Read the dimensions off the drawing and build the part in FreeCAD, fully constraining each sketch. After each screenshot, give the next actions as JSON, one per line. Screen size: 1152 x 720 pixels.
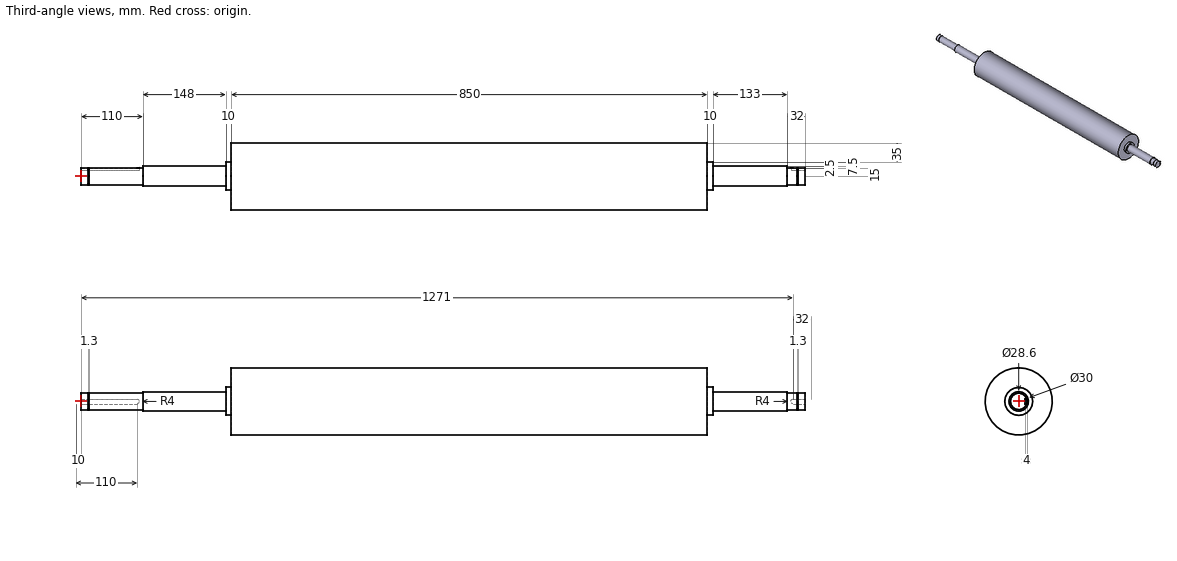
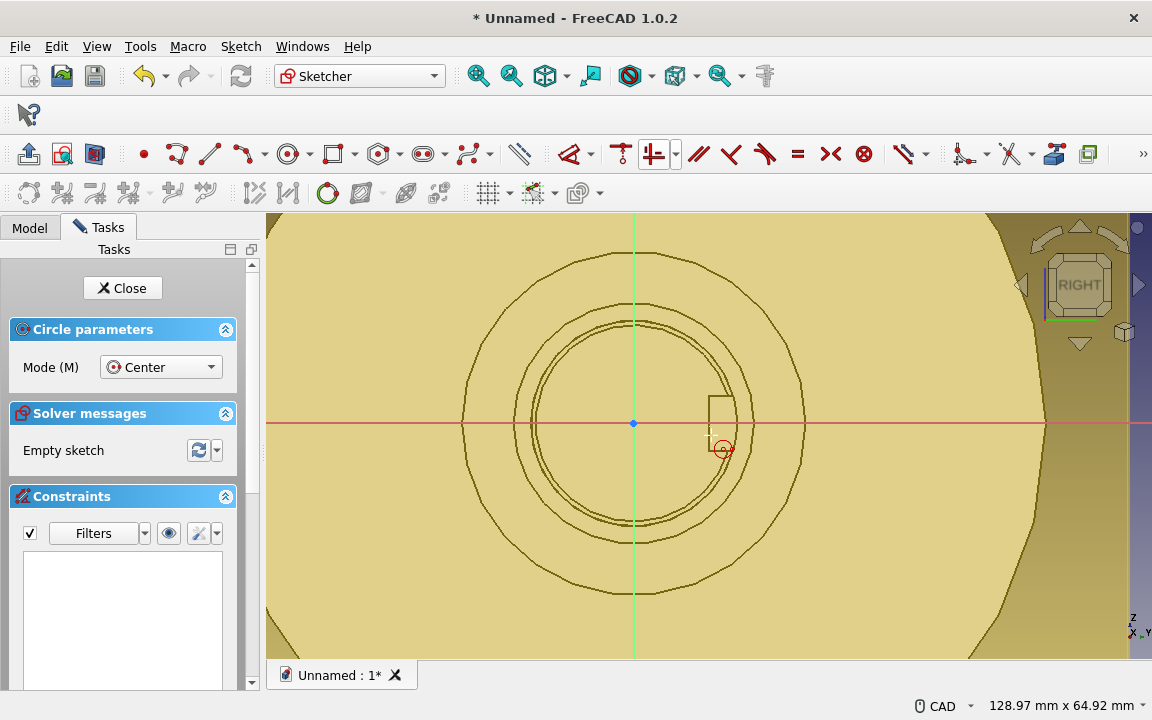
{"action": "left_click", "coordinate": [634, 423]}
{"action": "mouse_move", "coordinate": [707, 351]}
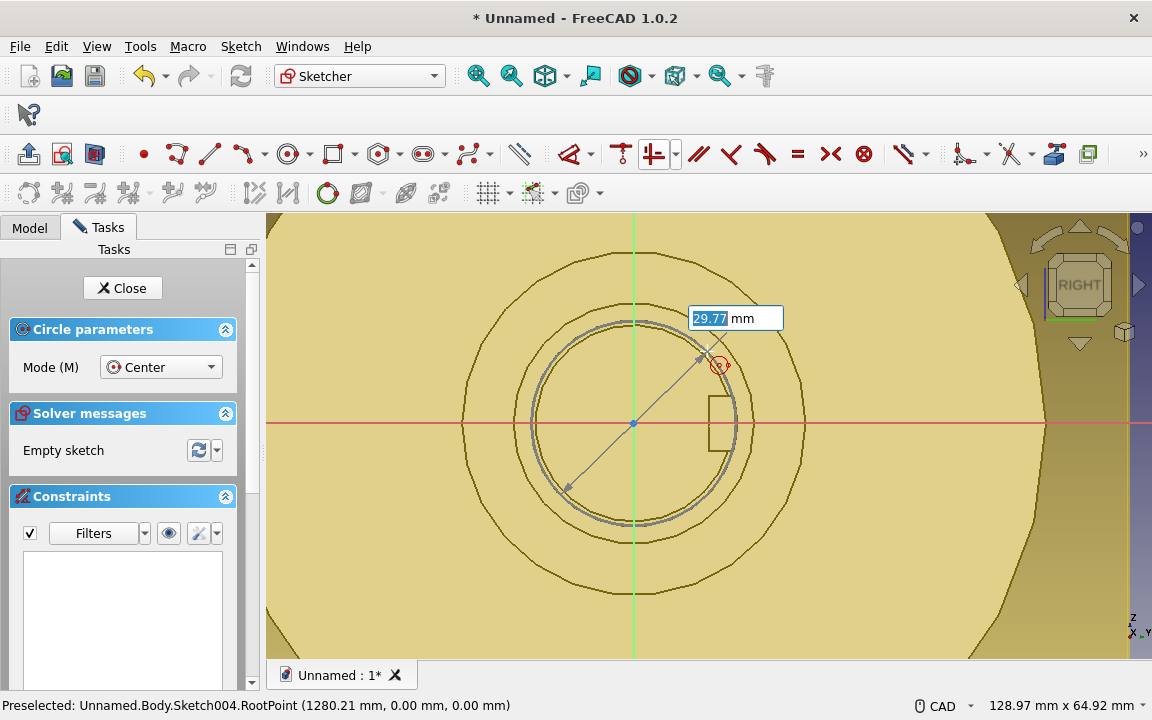
{"action": "type", "text": "30"}
{"action": "key", "text": "Return"}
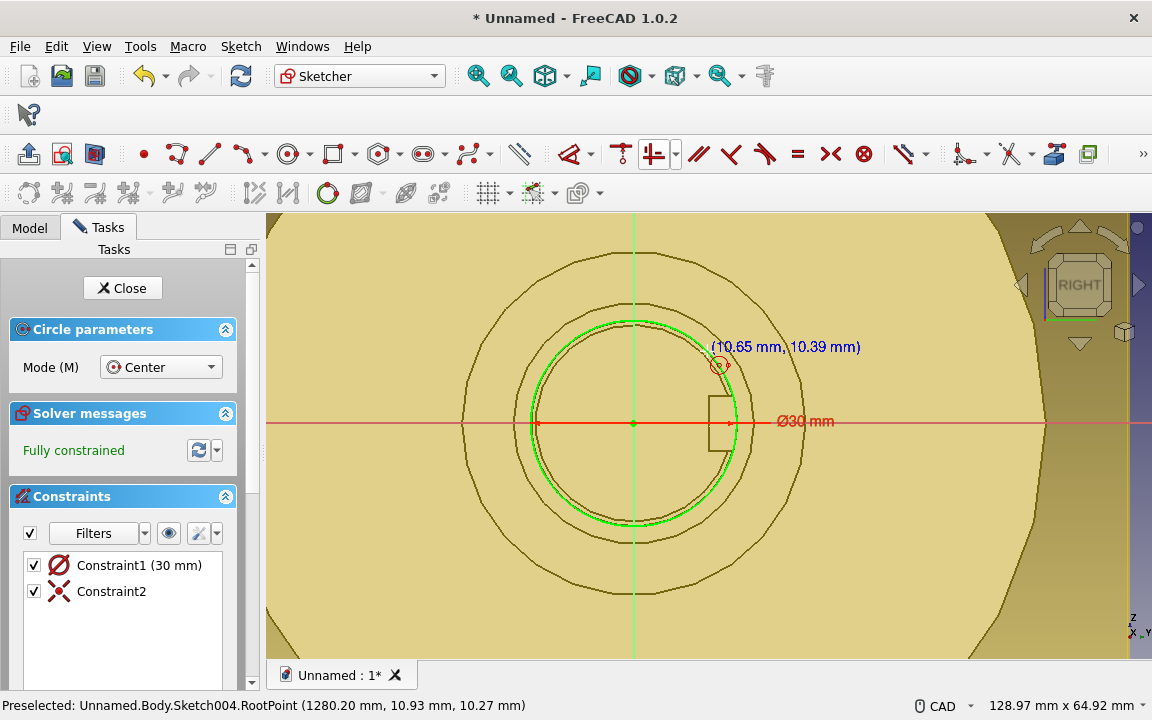
{"action": "left_click", "coordinate": [634, 423]}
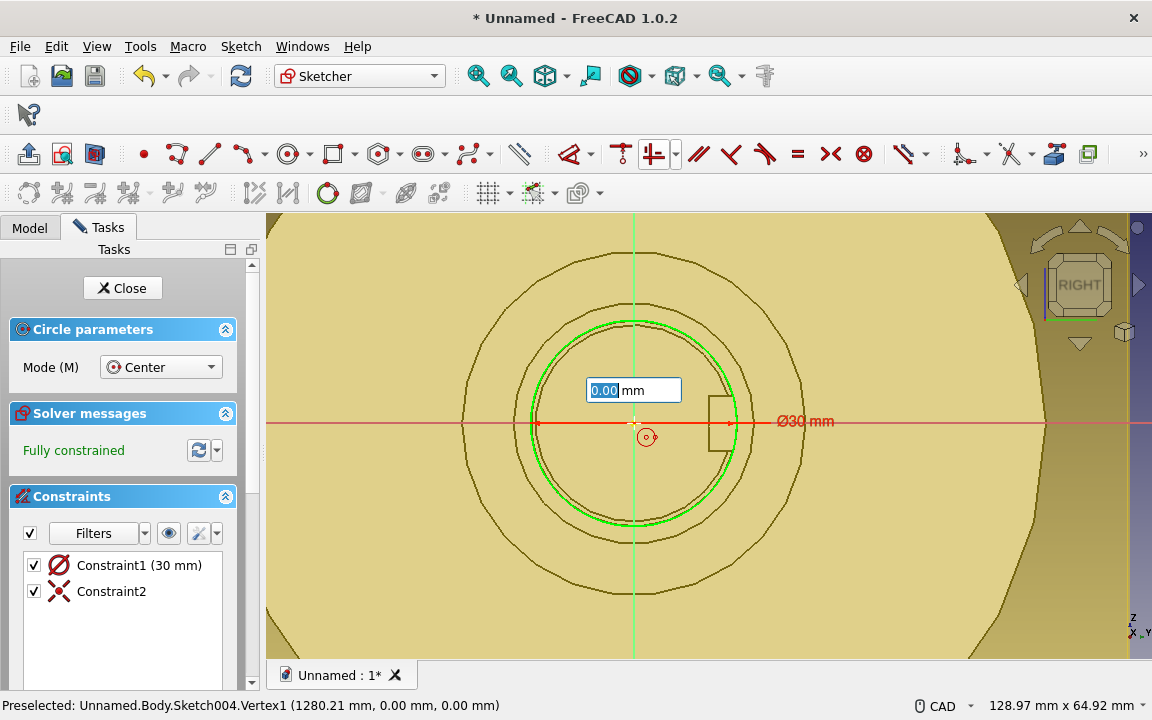
{"action": "scroll", "coordinate": [667, 331], "scroll_direction": "up", "scroll_amount": 6}
{"action": "mouse_move", "coordinate": [667, 331]}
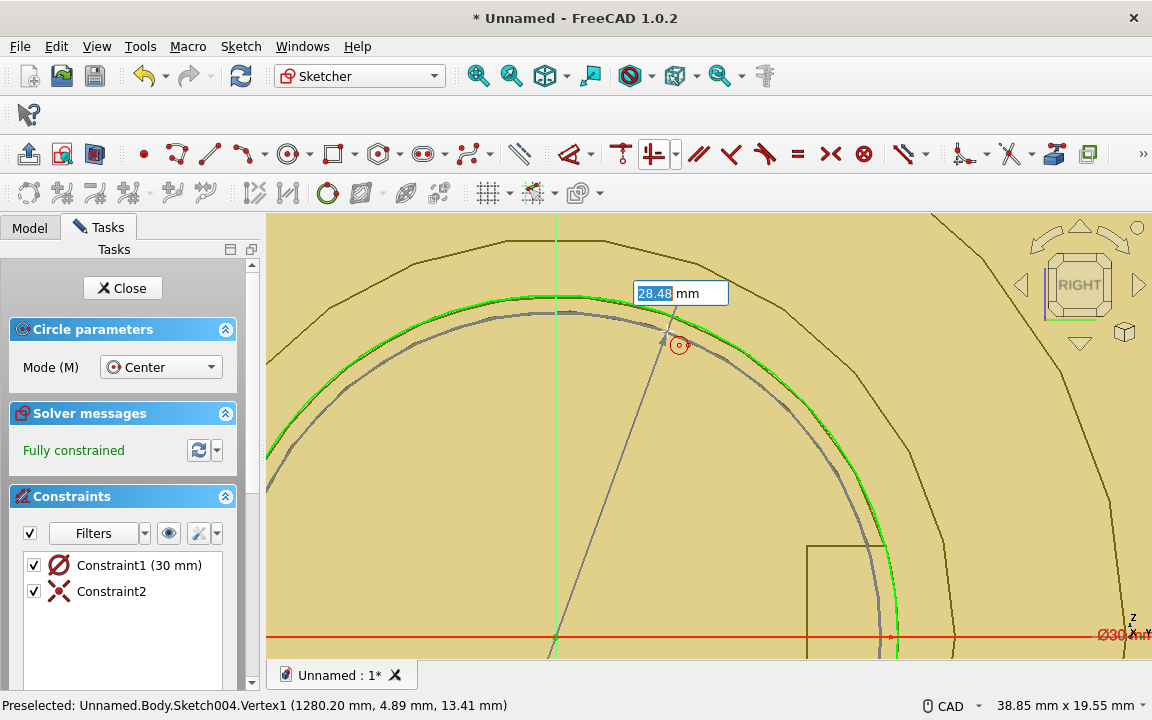
{"action": "type", "text": "28.6"}
{"action": "key", "text": "Return"}
{"action": "key", "text": "Escape"}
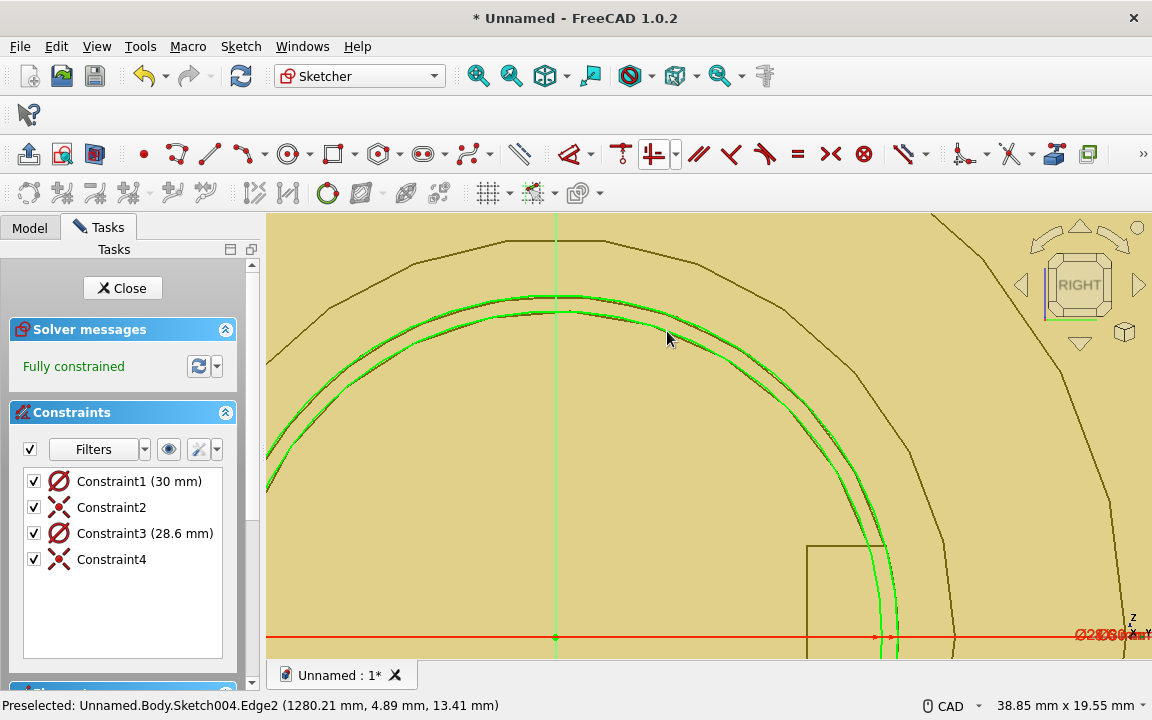
{"action": "left_click", "coordinate": [123, 288]}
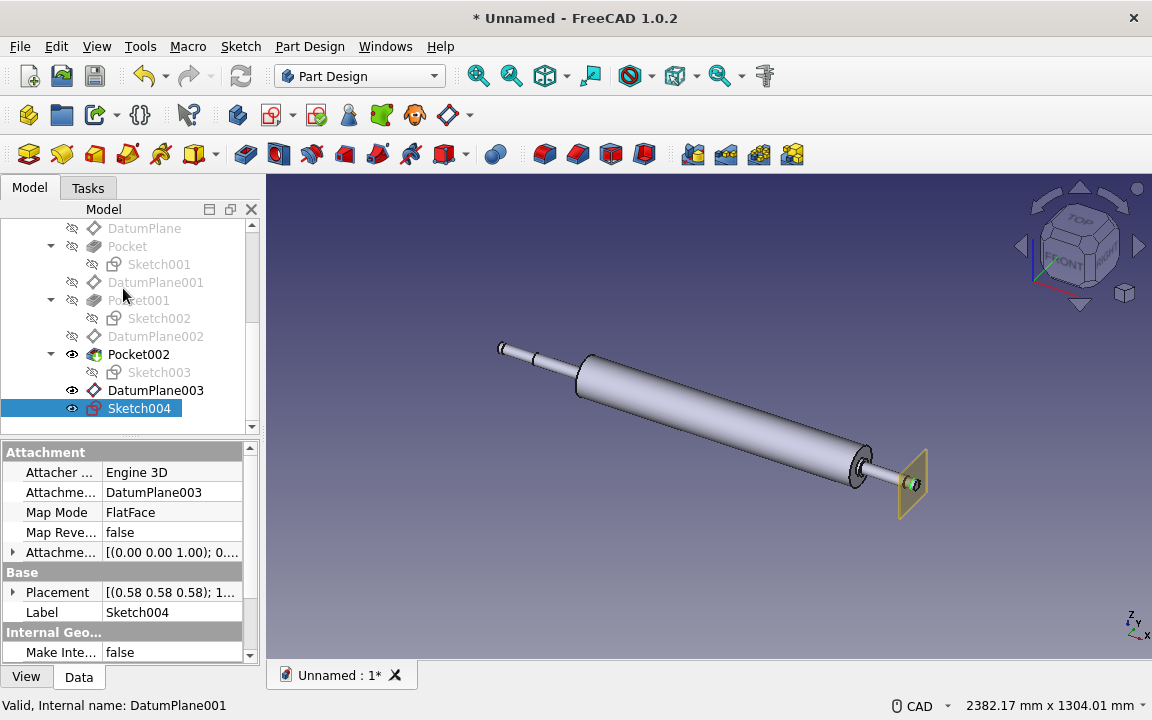
{"action": "left_click", "coordinate": [246, 154]}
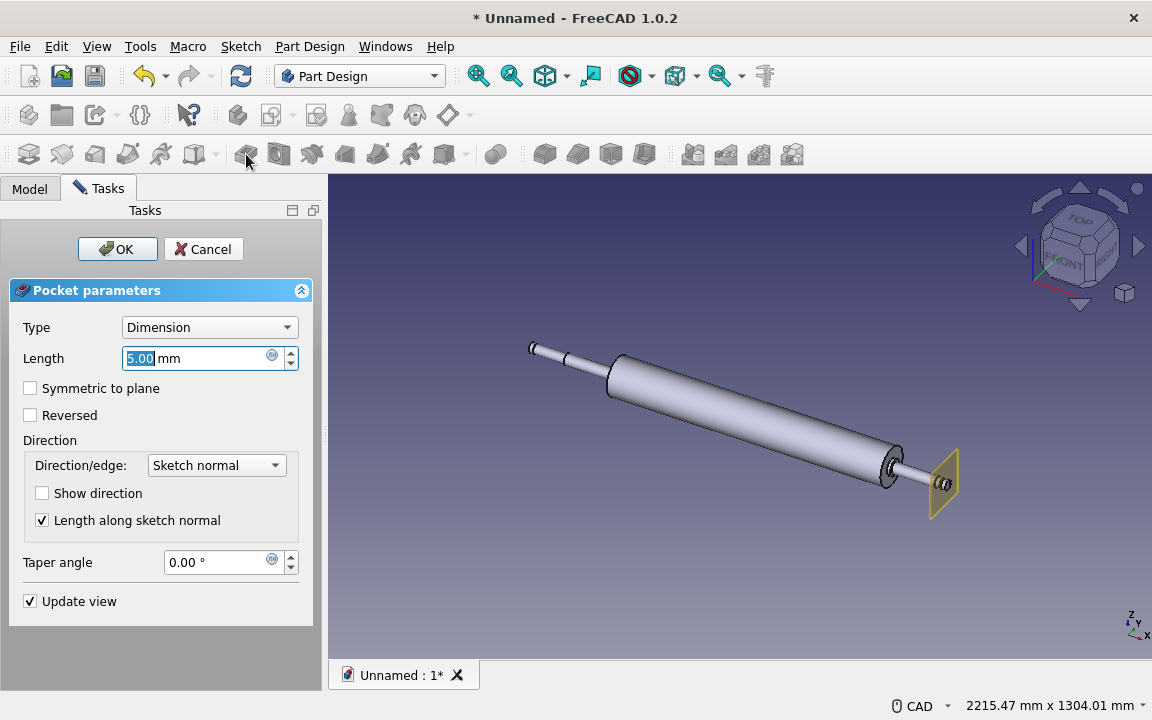
{"action": "type", "text": "1.3"}
{"action": "key", "text": "Tab"}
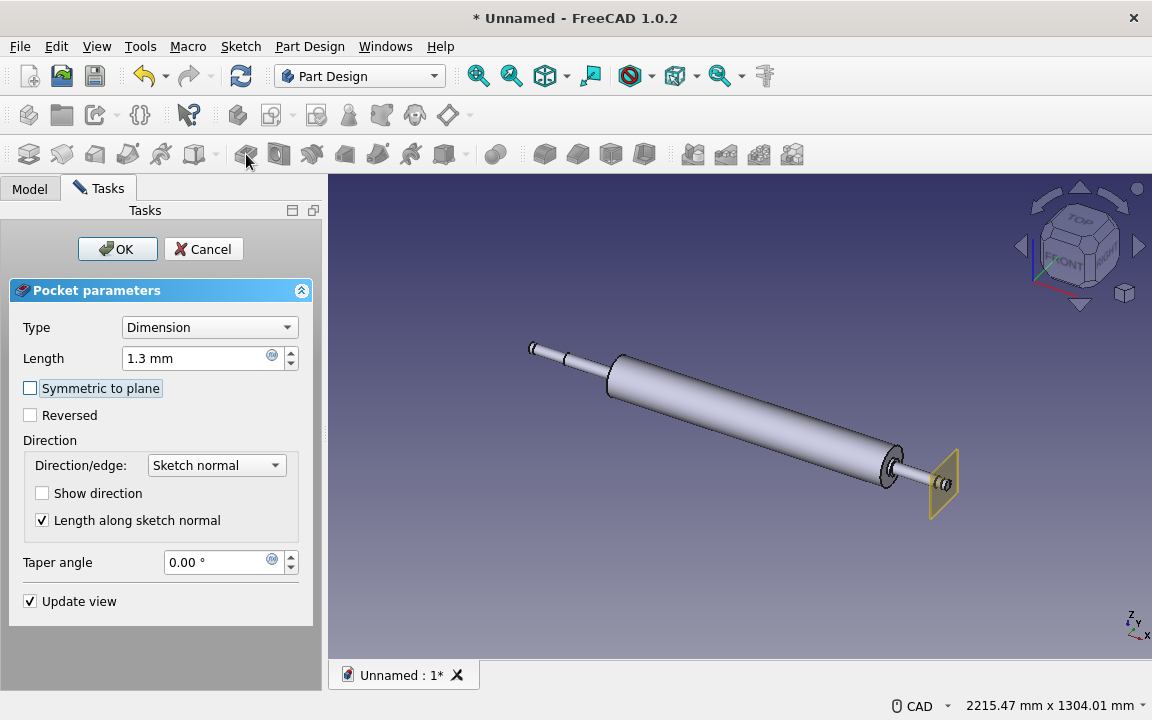
{"action": "left_click", "coordinate": [118, 249]}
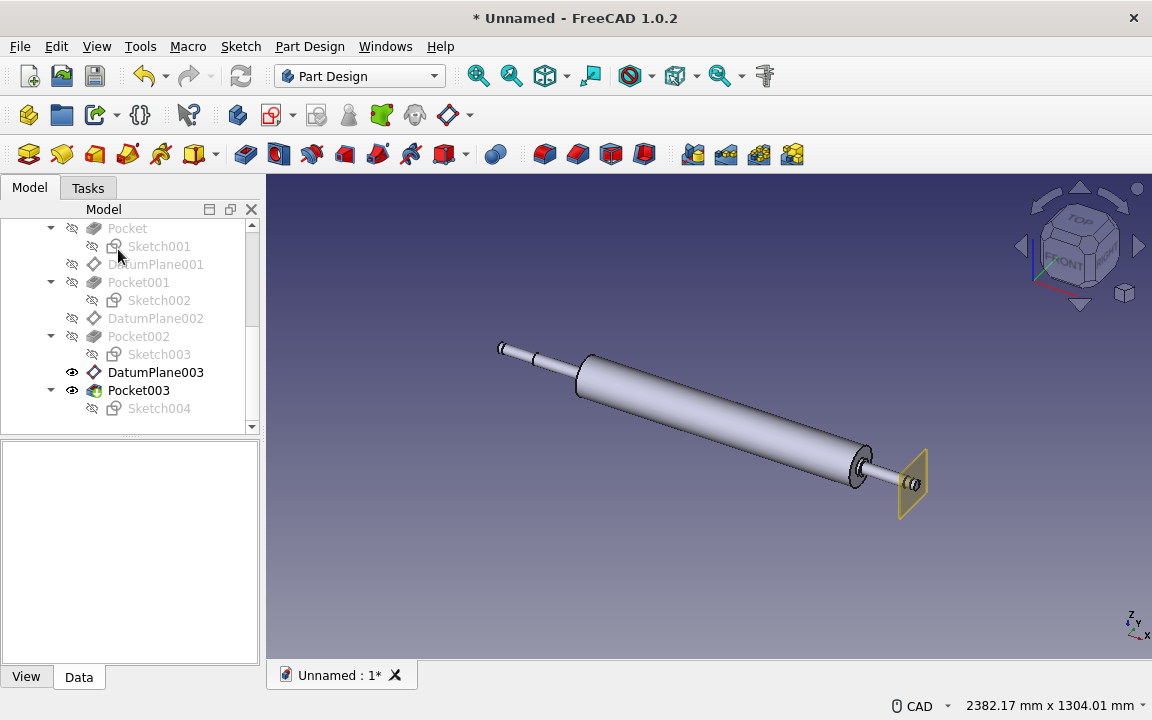
{"action": "left_click", "coordinate": [117, 372]}
{"action": "key", "text": "space"}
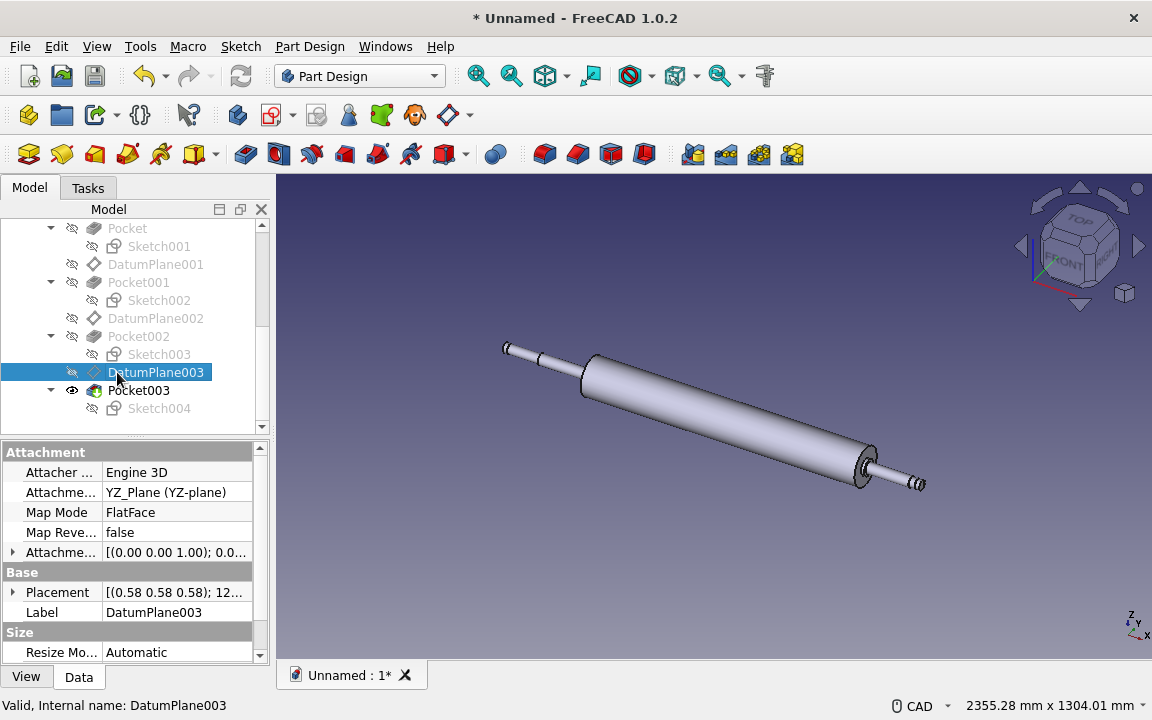
{"action": "key", "text": "0"}